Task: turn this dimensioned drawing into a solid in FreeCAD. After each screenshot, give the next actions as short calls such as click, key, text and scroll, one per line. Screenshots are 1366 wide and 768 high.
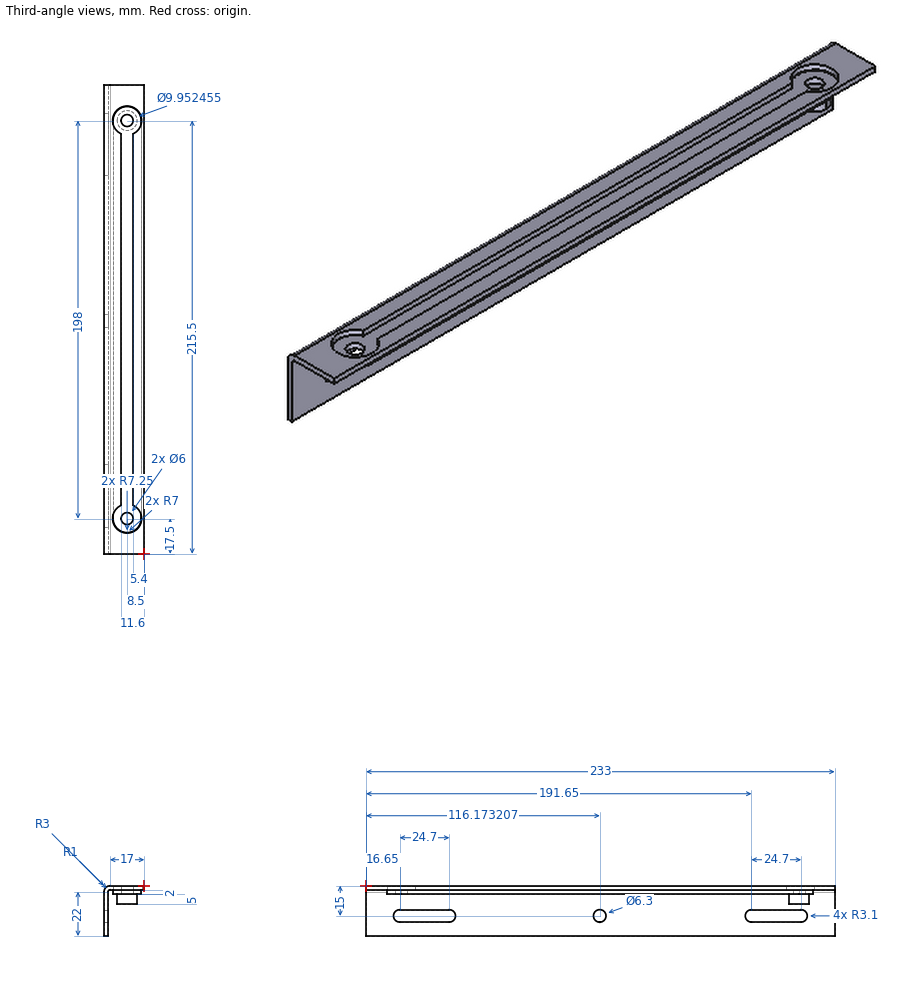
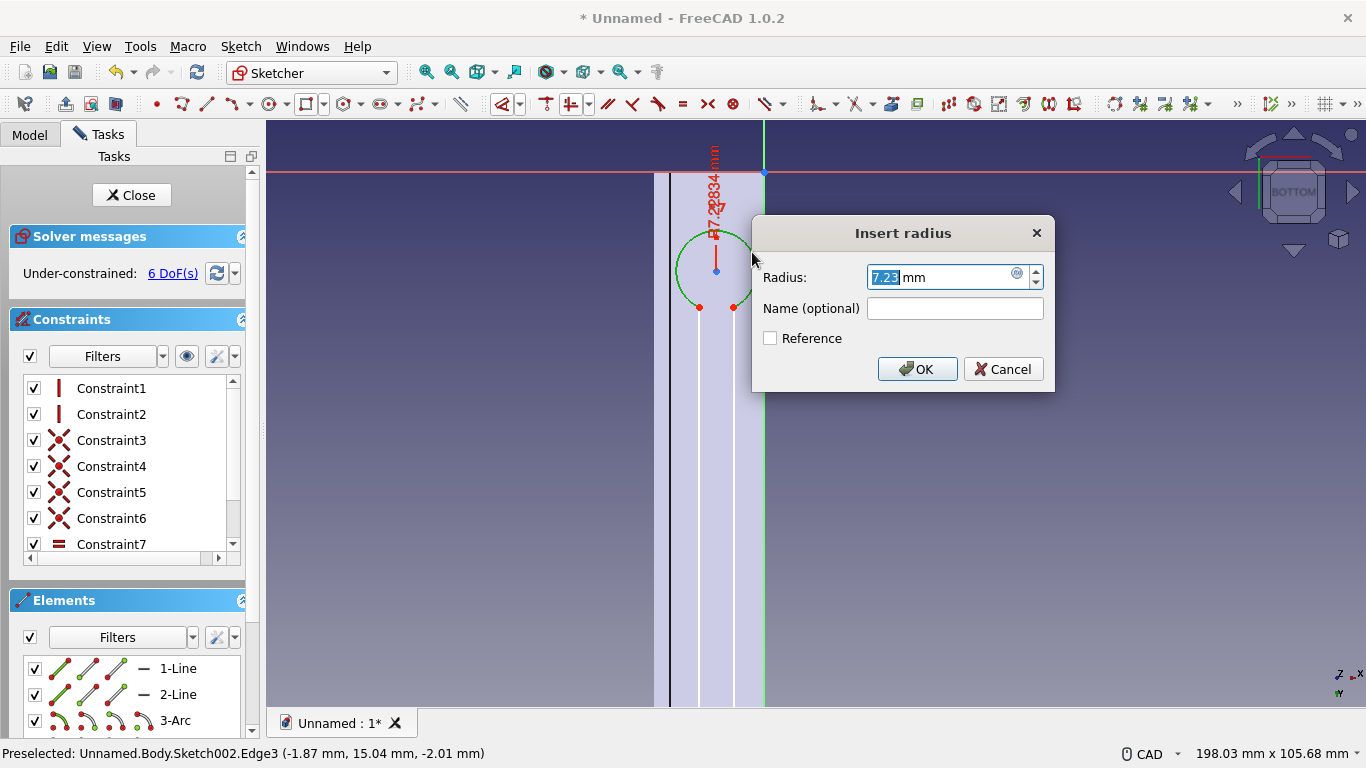
text(7.25)
key(Return)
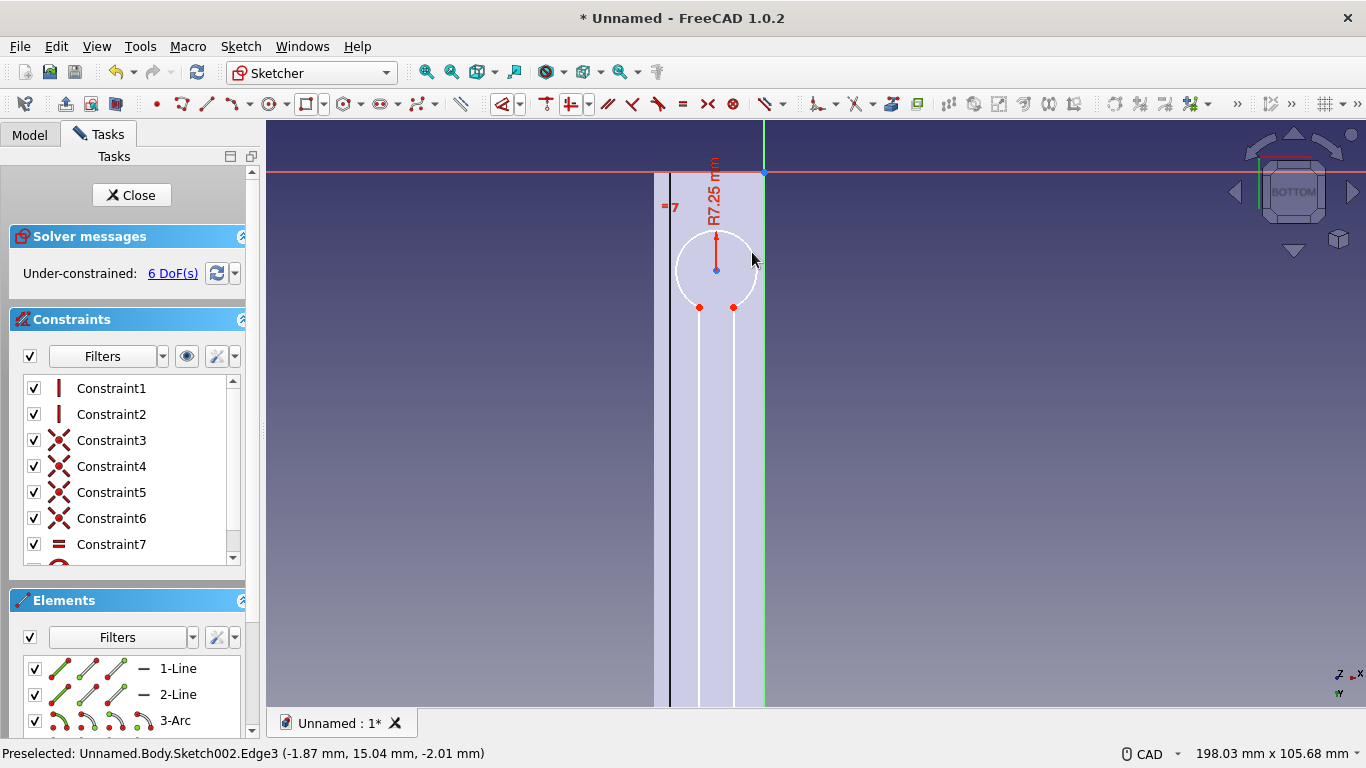
scroll(754, 251, down, 6)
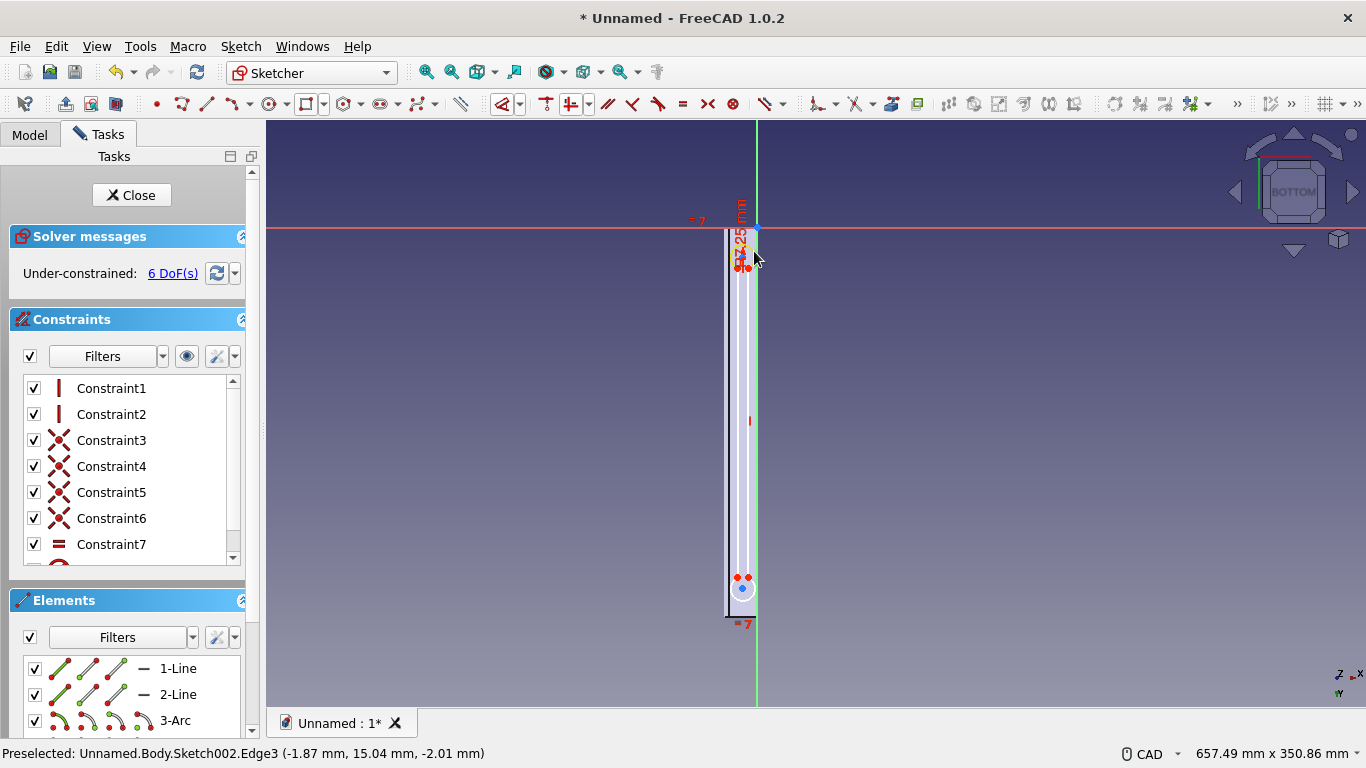
scroll(748, 578, up, 8)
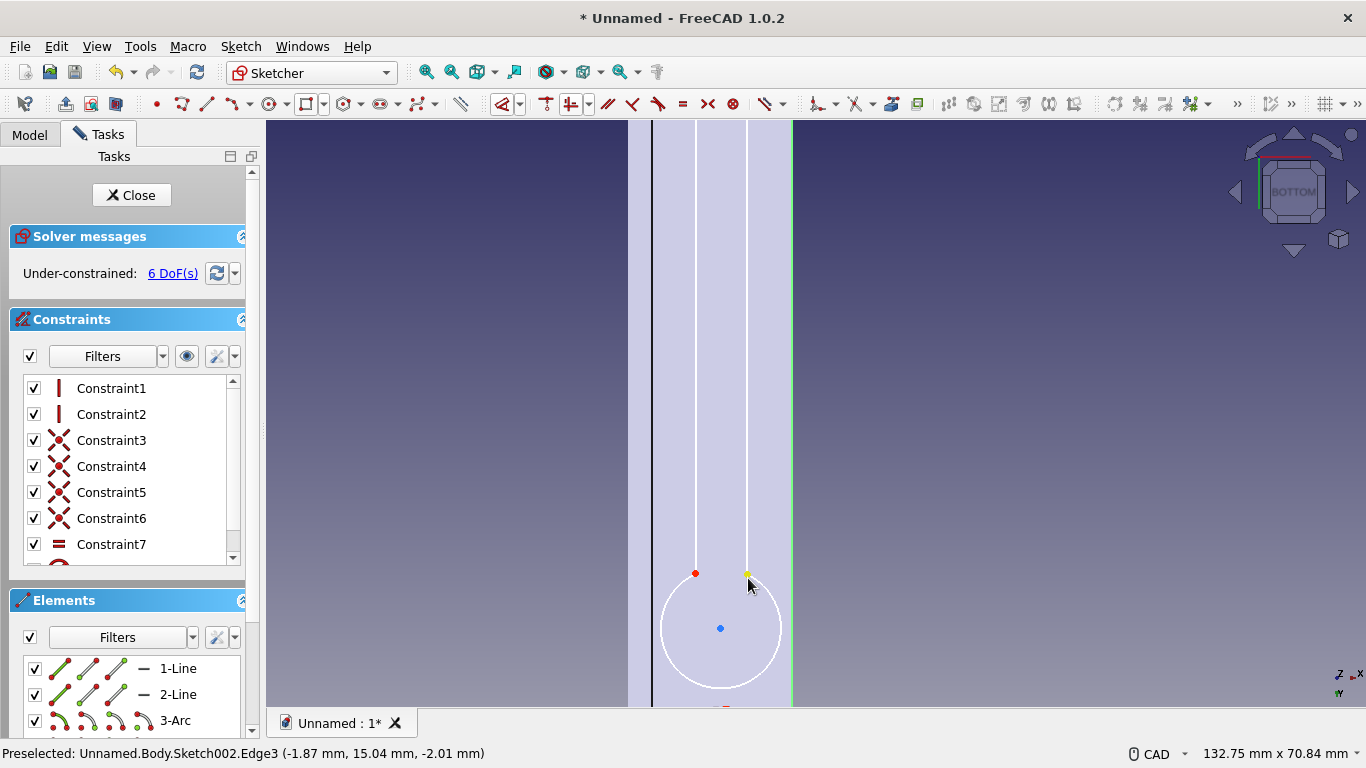
click(747, 574)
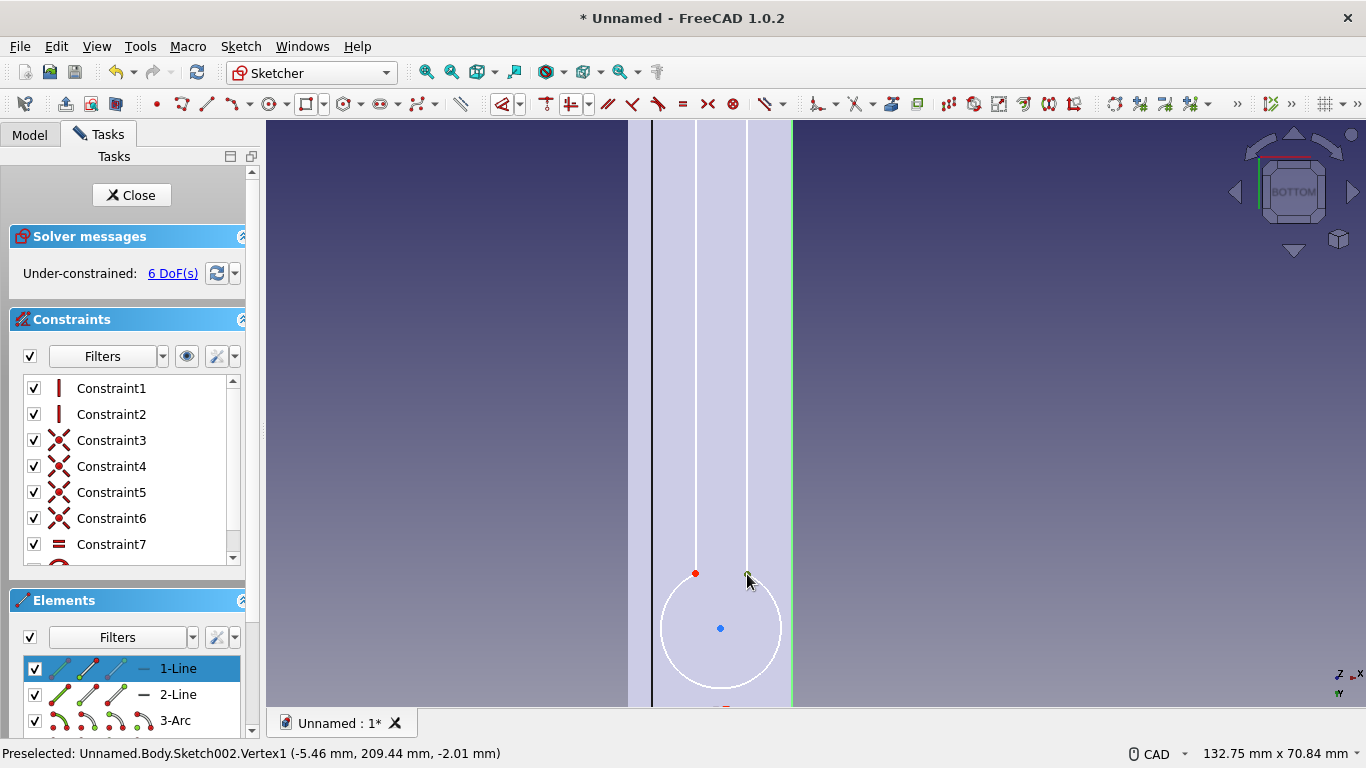
click(520, 104)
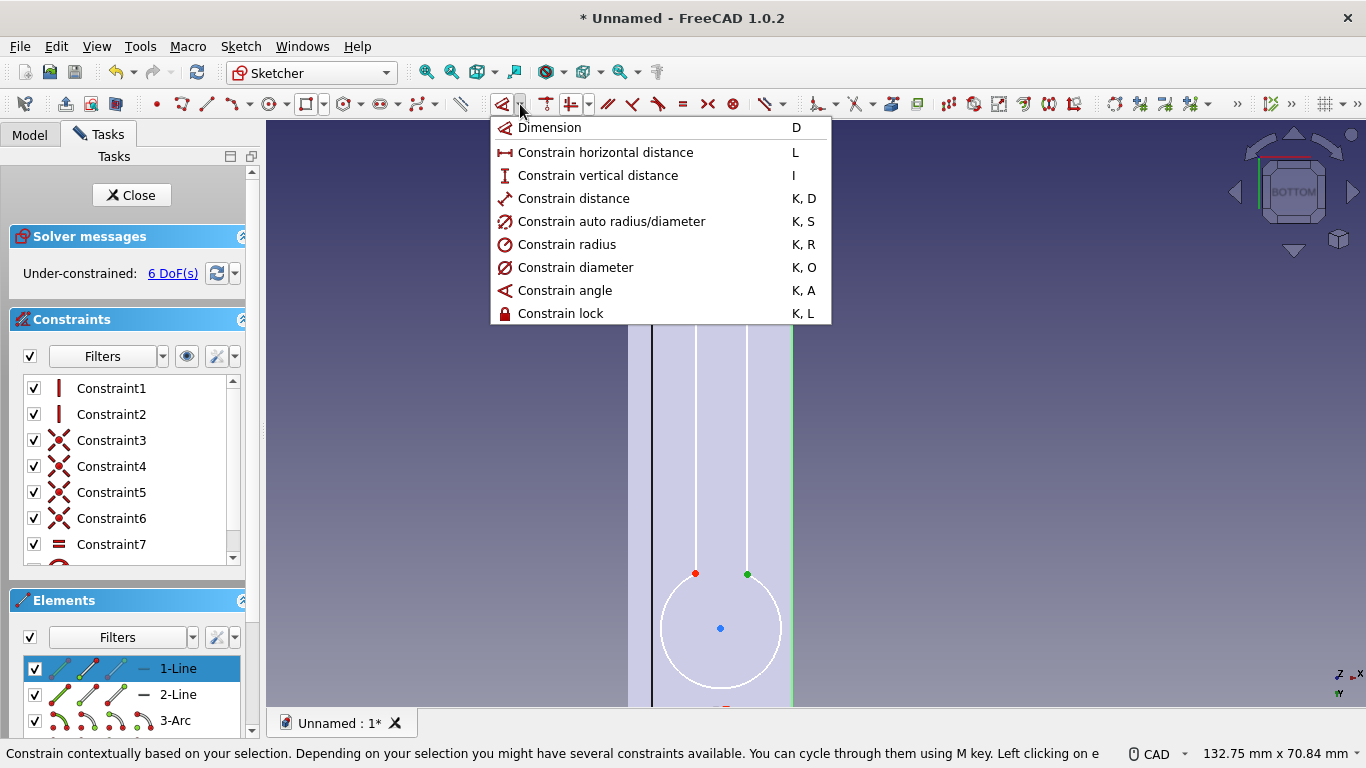
click(661, 152)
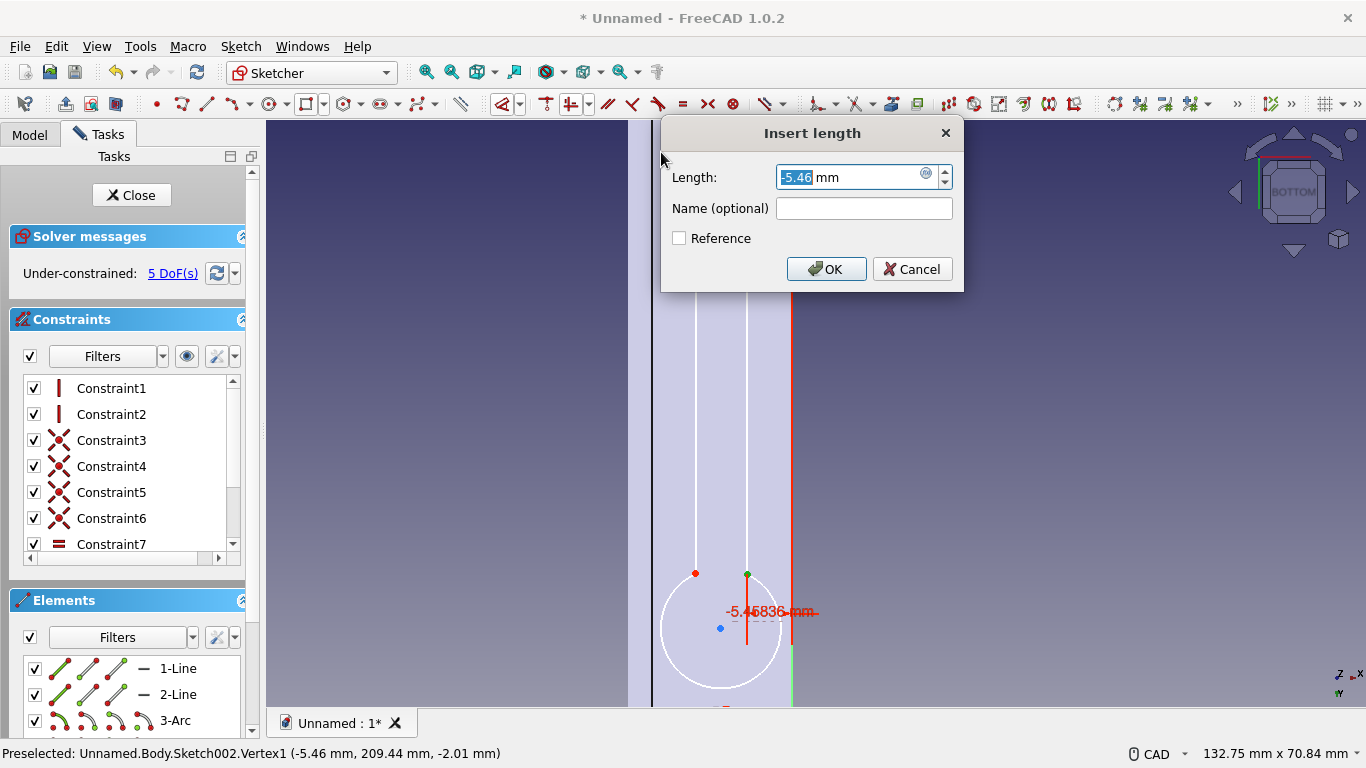
text(-5.4)
key(Return)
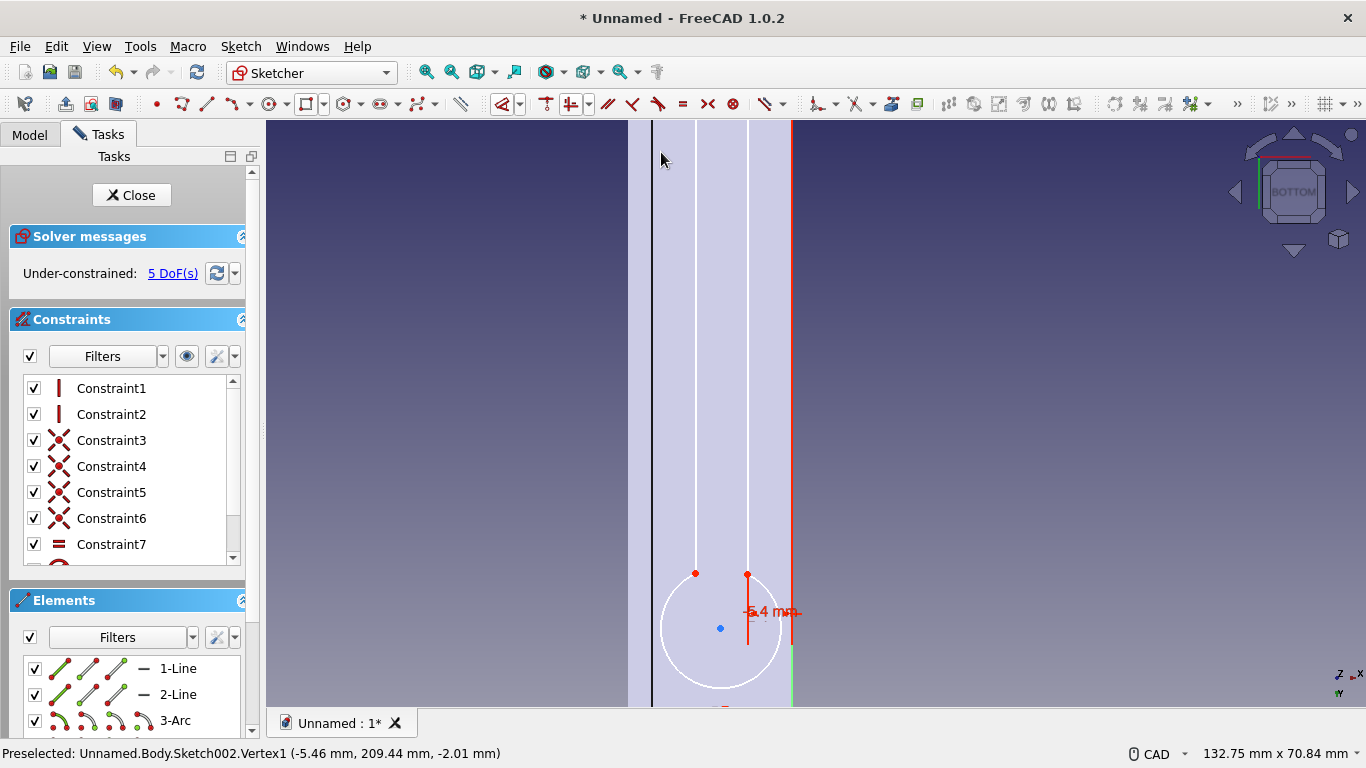
scroll(748, 578, down, 8)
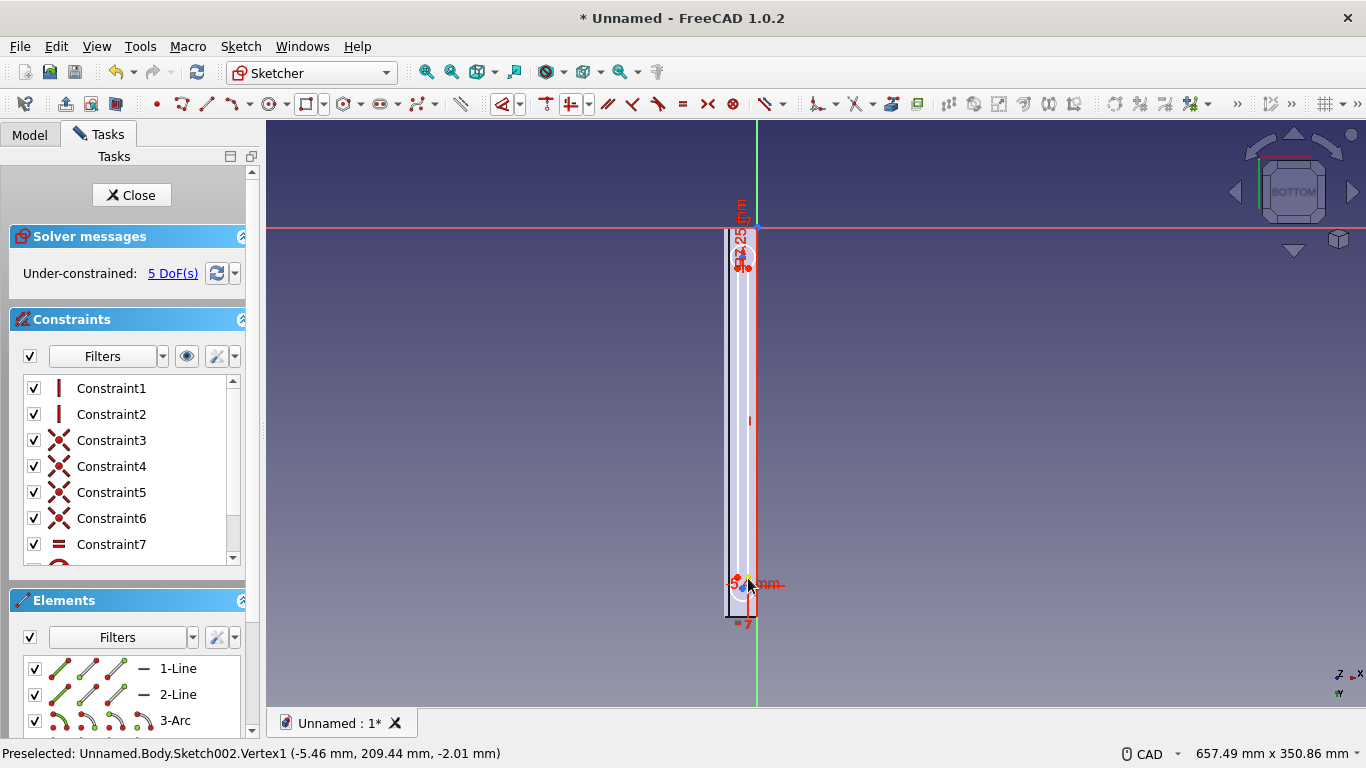
scroll(743, 257, up, 6)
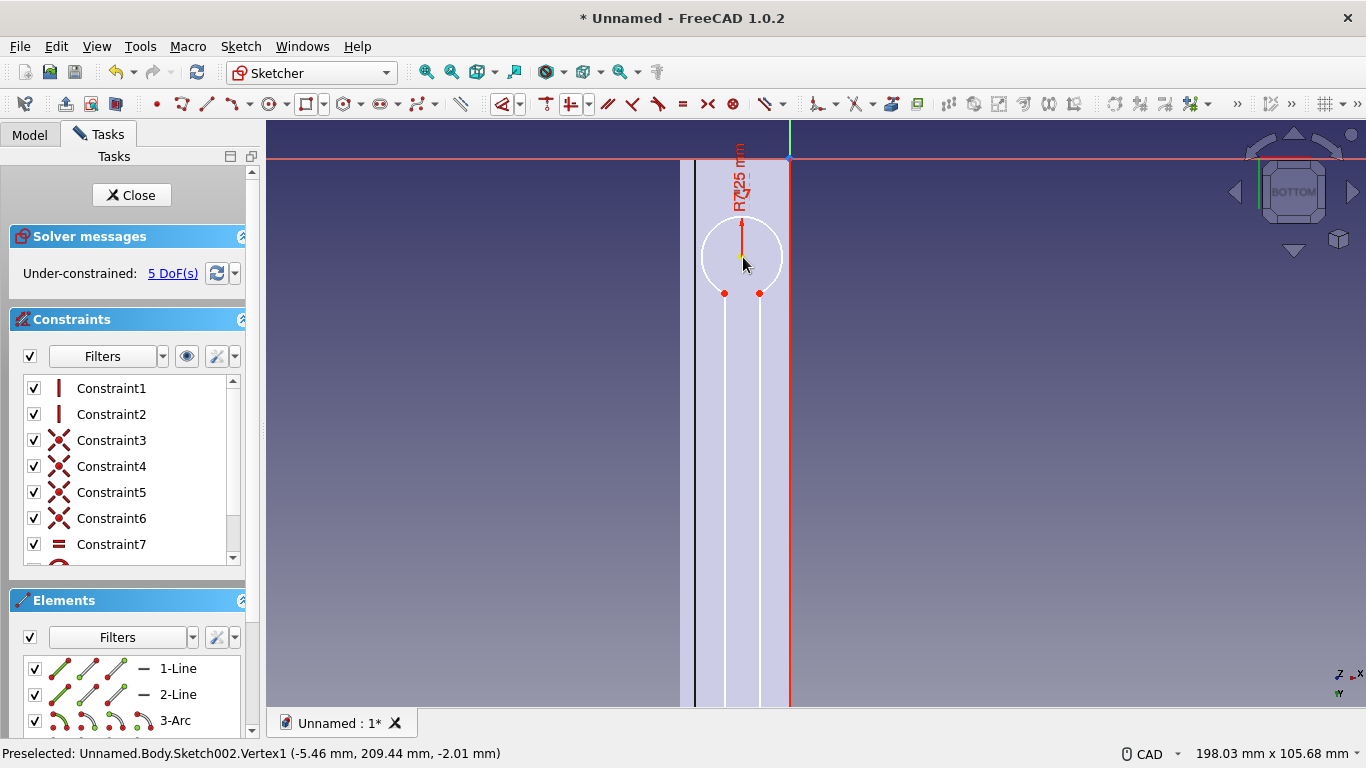
click(742, 257)